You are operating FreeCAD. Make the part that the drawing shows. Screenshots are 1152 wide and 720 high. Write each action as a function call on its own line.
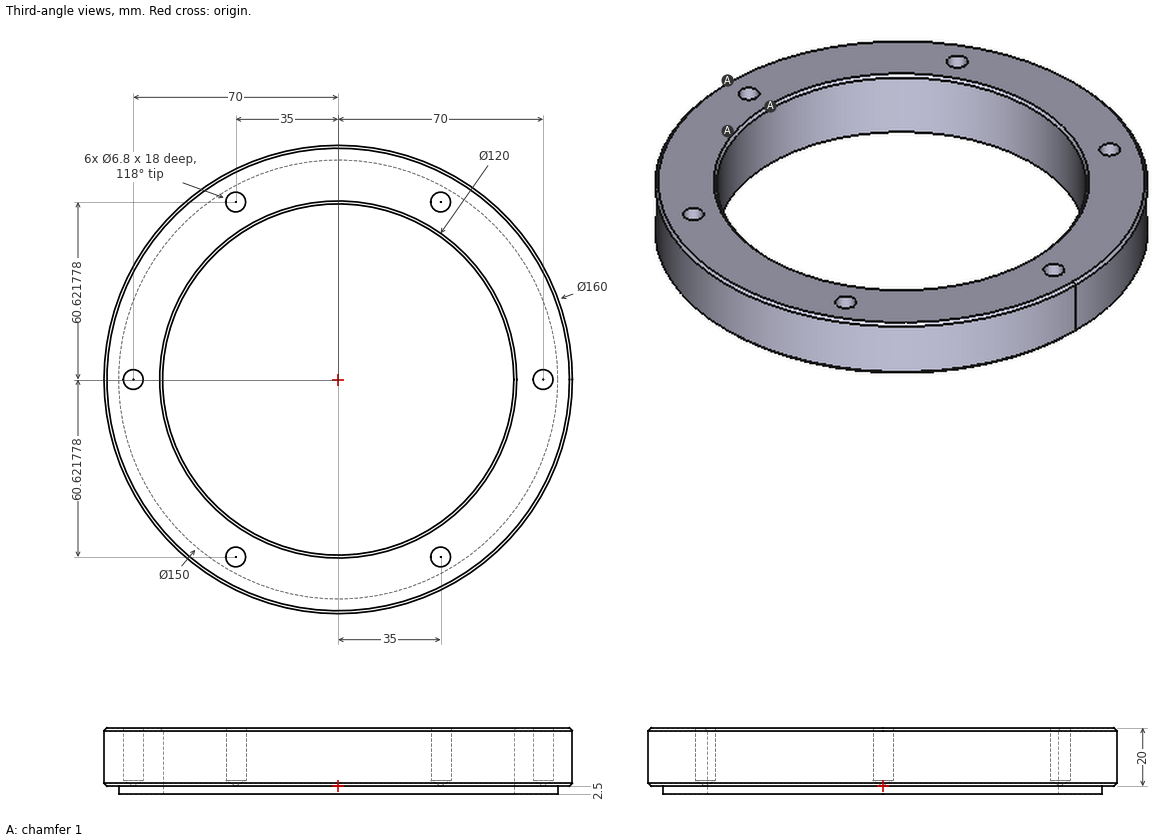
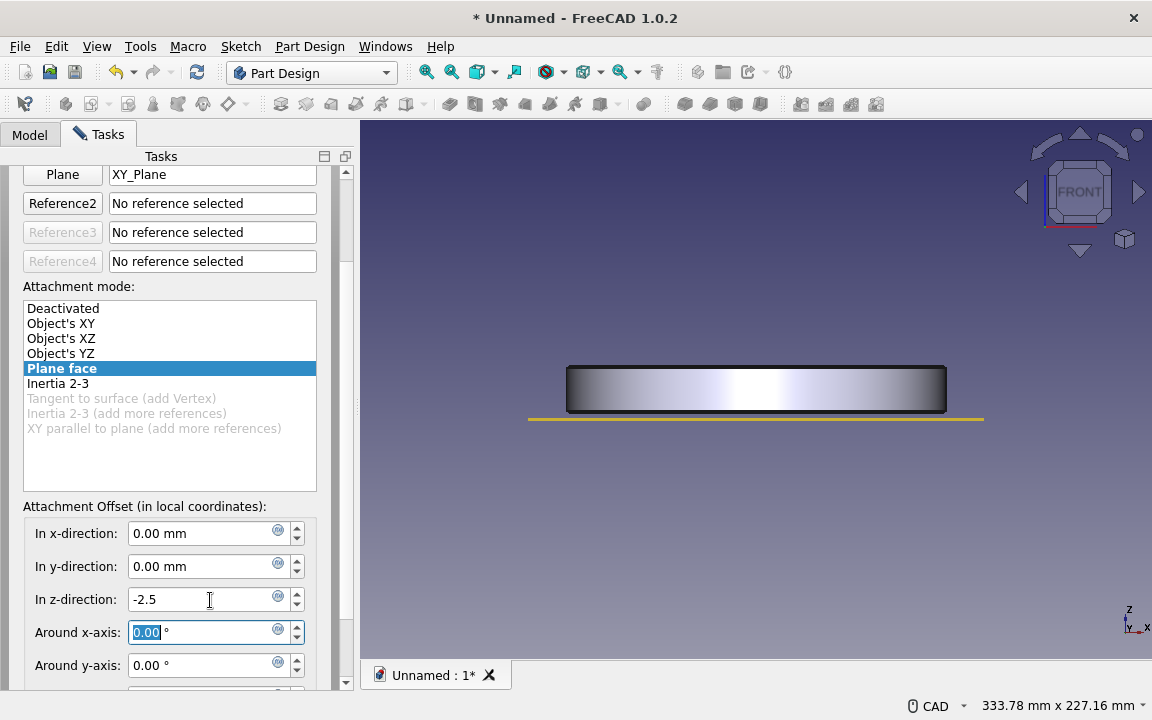
scroll(346, 428, up, 3)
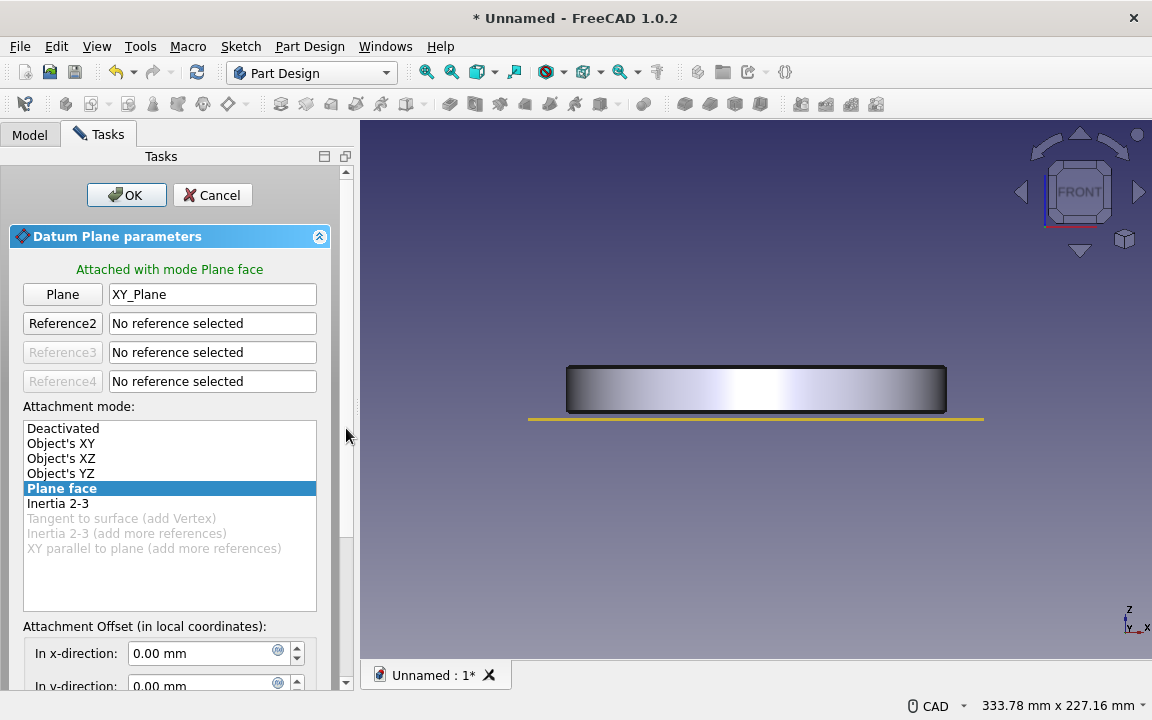
click(127, 195)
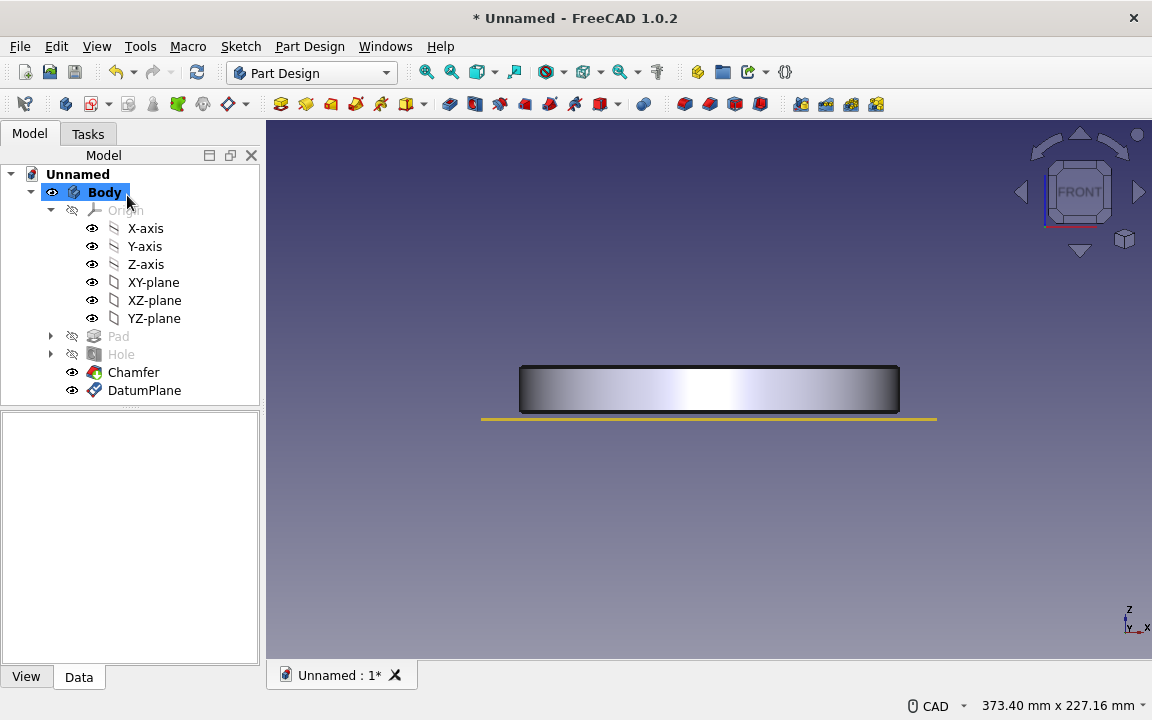
click(117, 390)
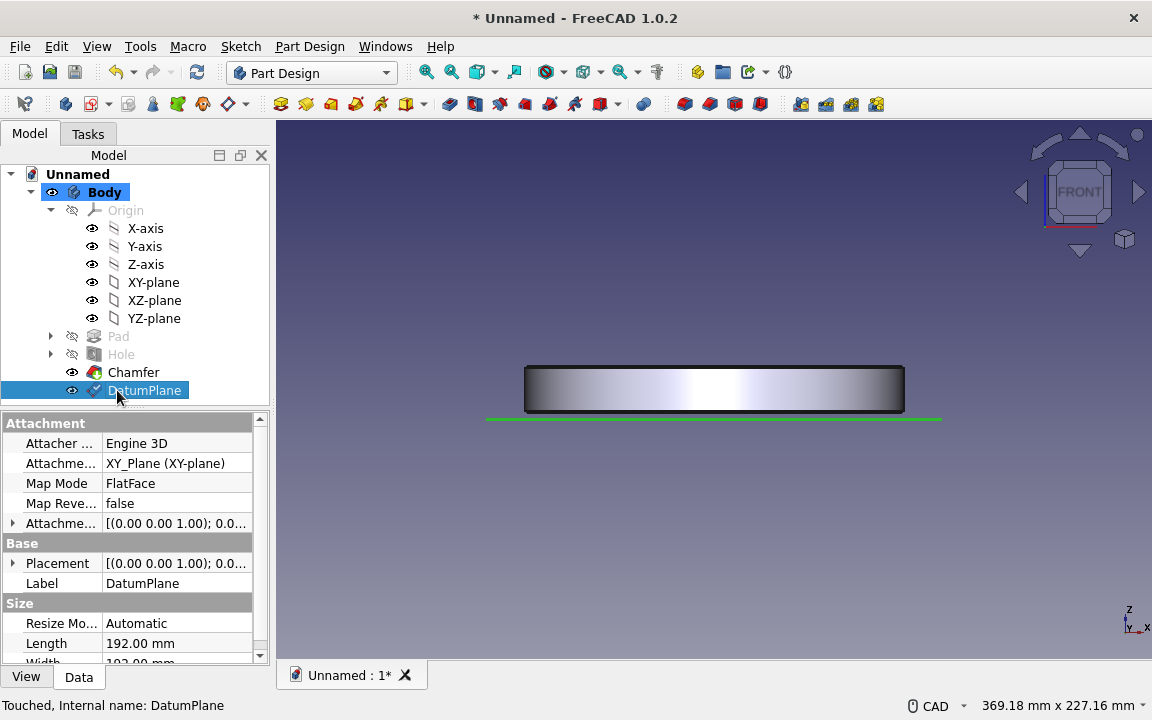
click(90, 104)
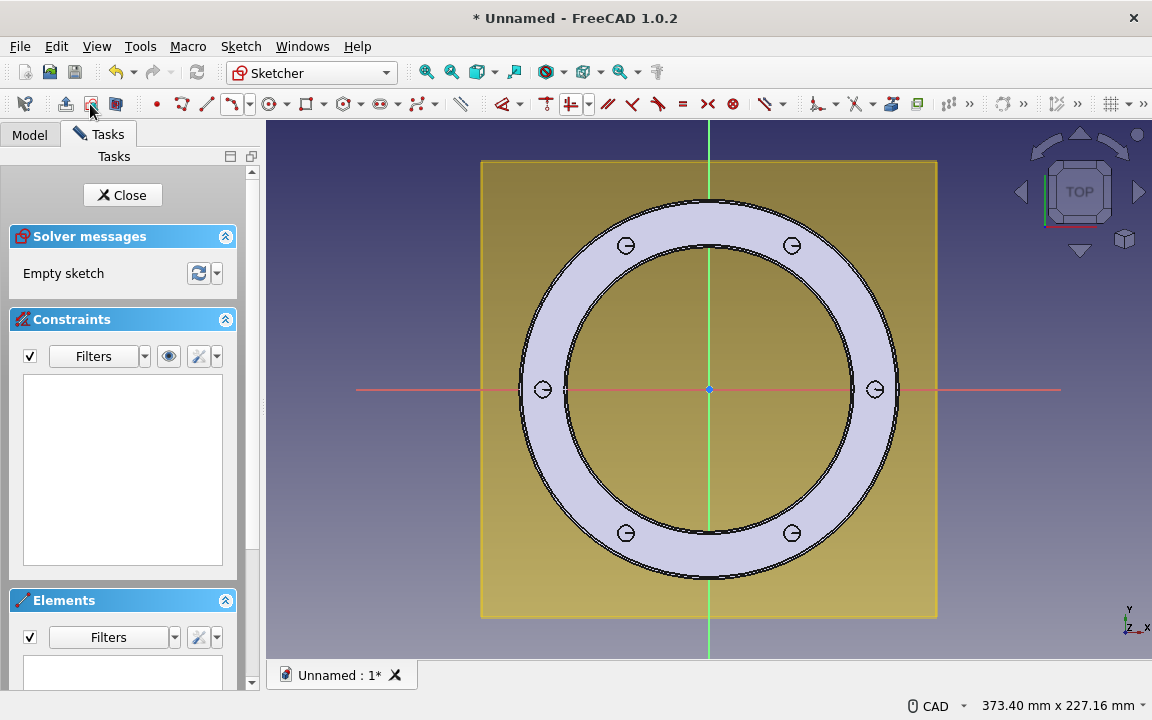
click(116, 104)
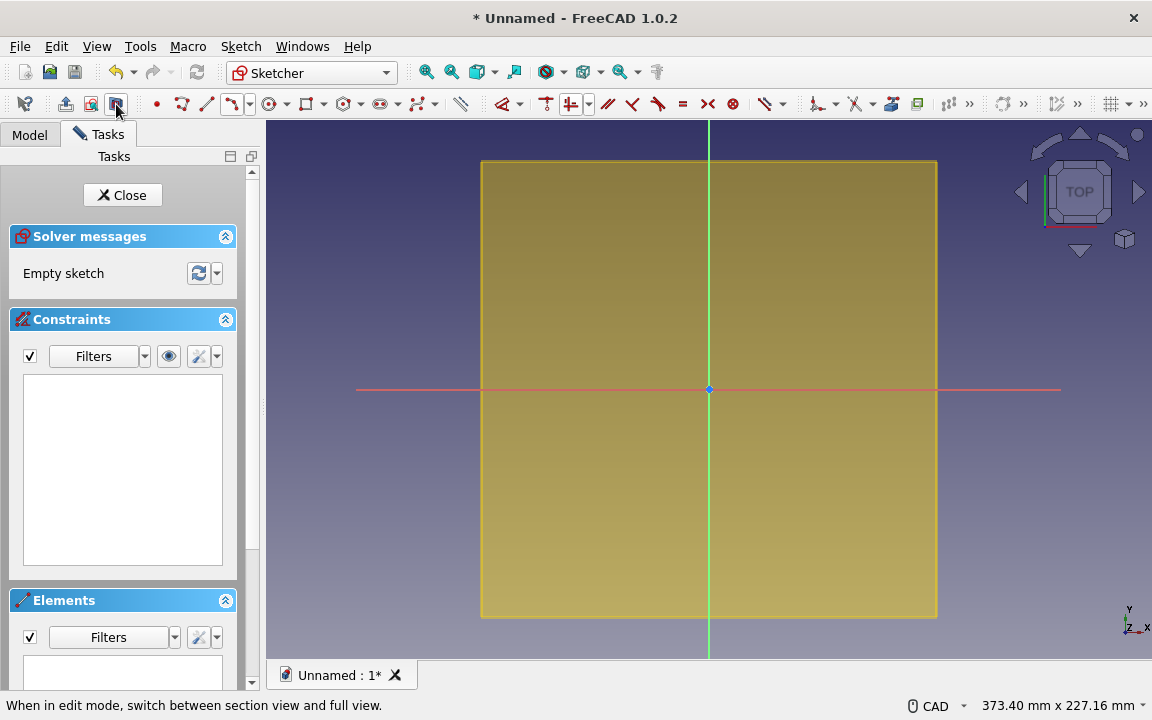
key(g)
key(c)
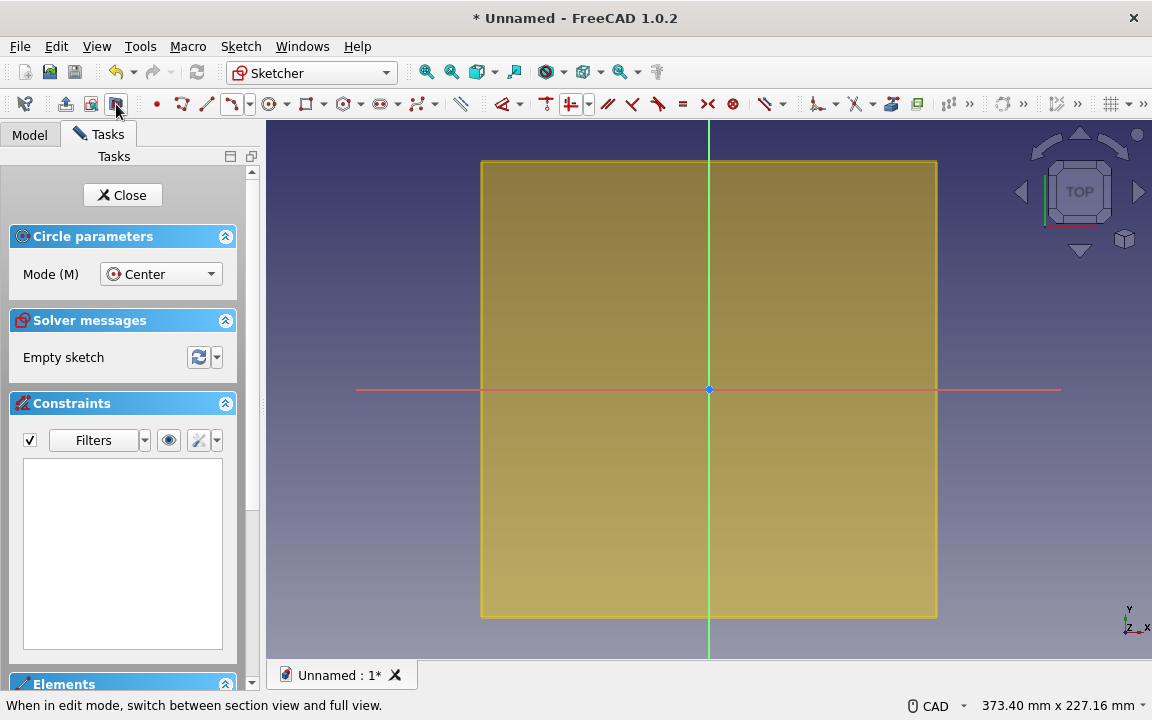
click(709, 390)
click(835, 264)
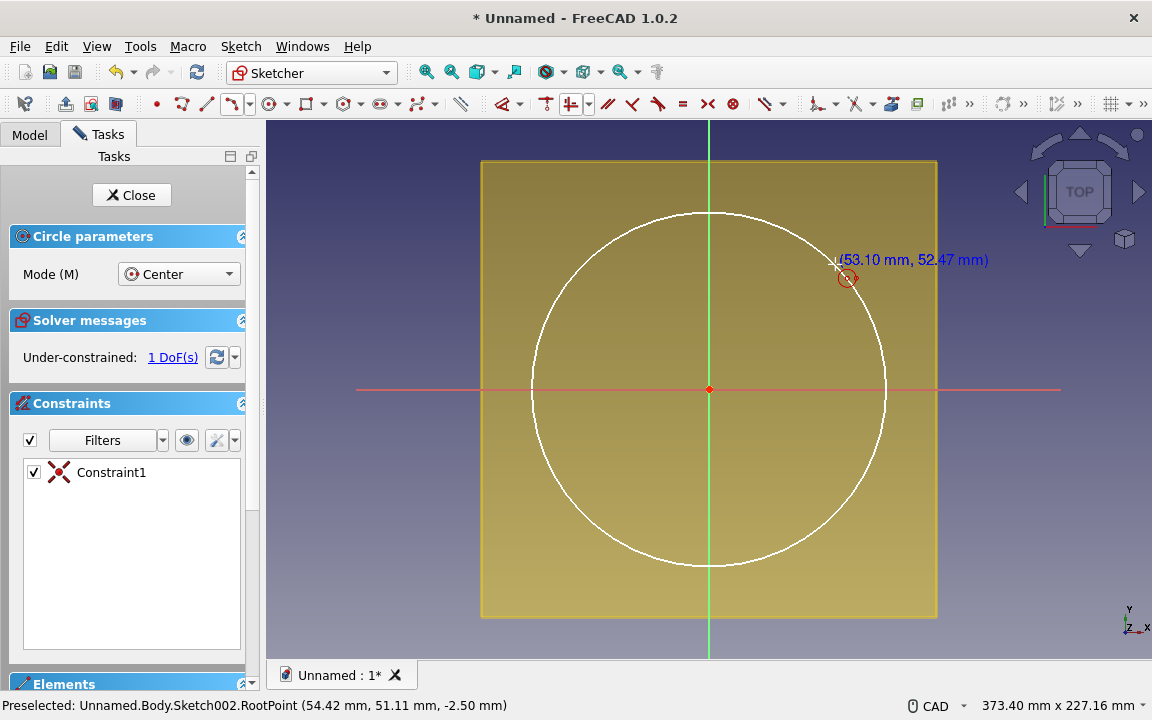
click(709, 390)
click(810, 289)
key(Escape)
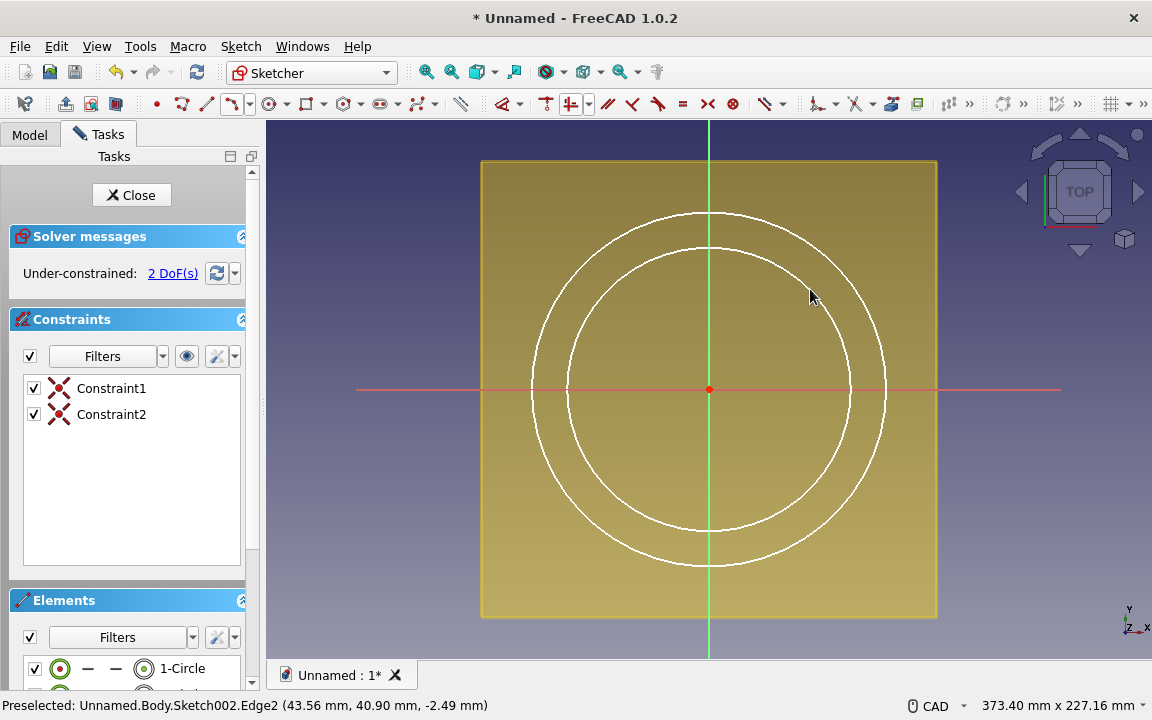
click(502, 104)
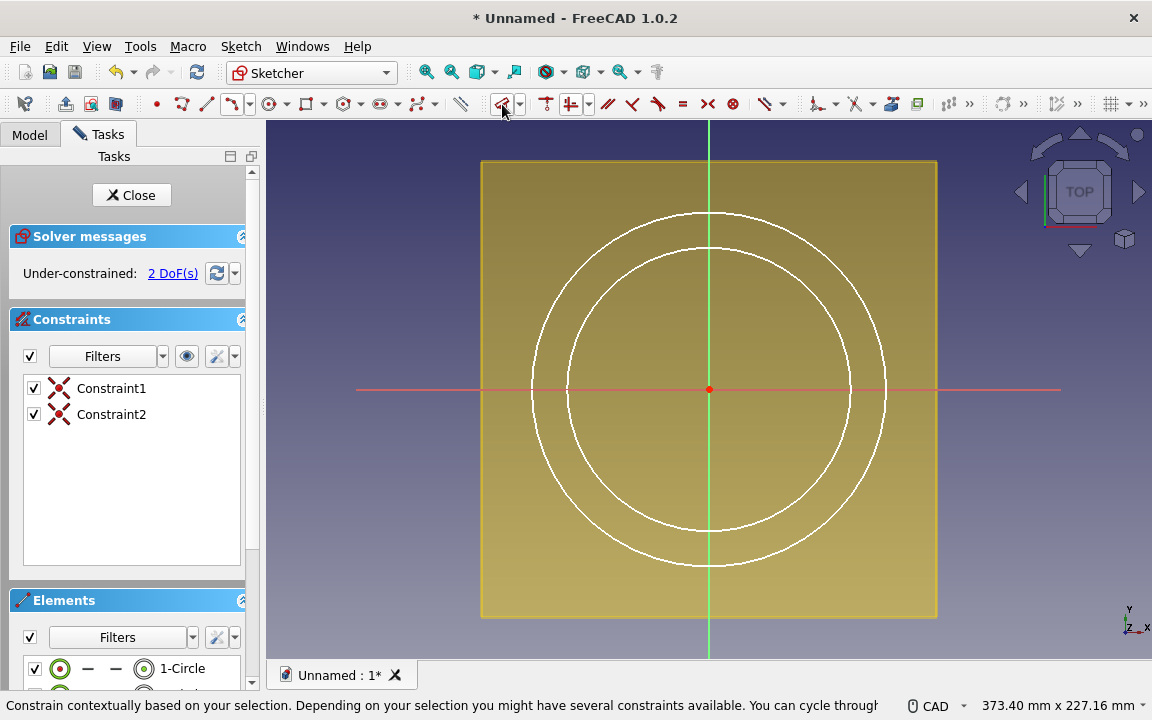
click(834, 264)
click(857, 241)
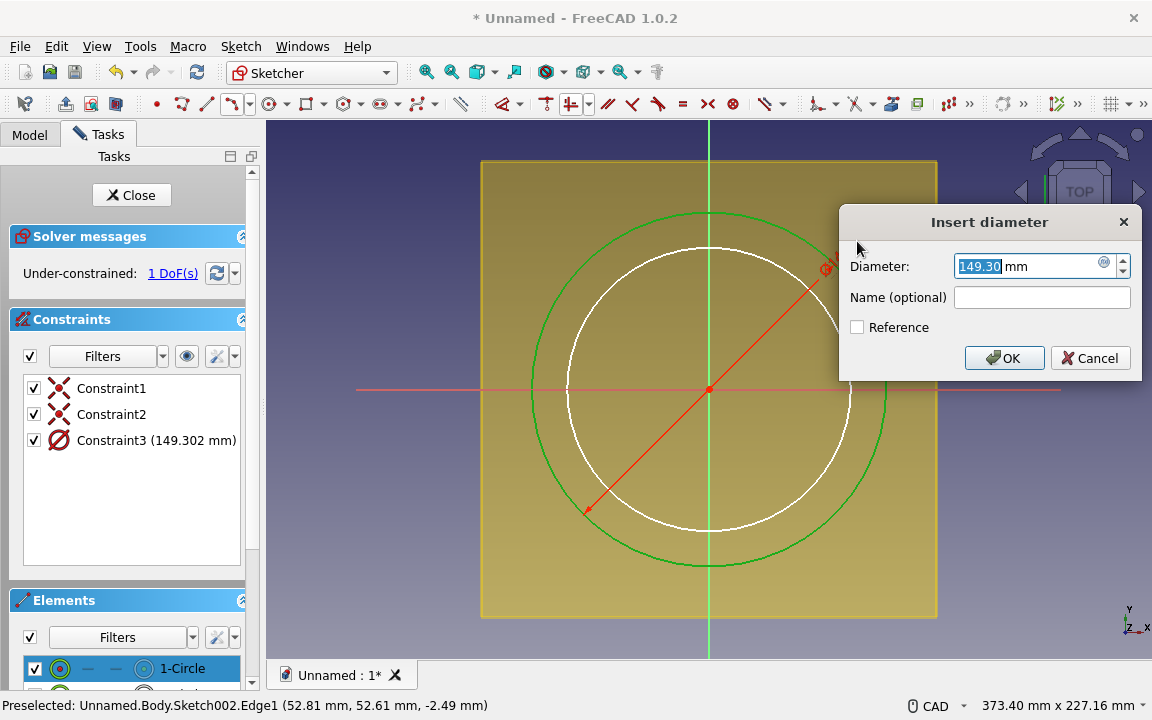
text(150)
key(Return)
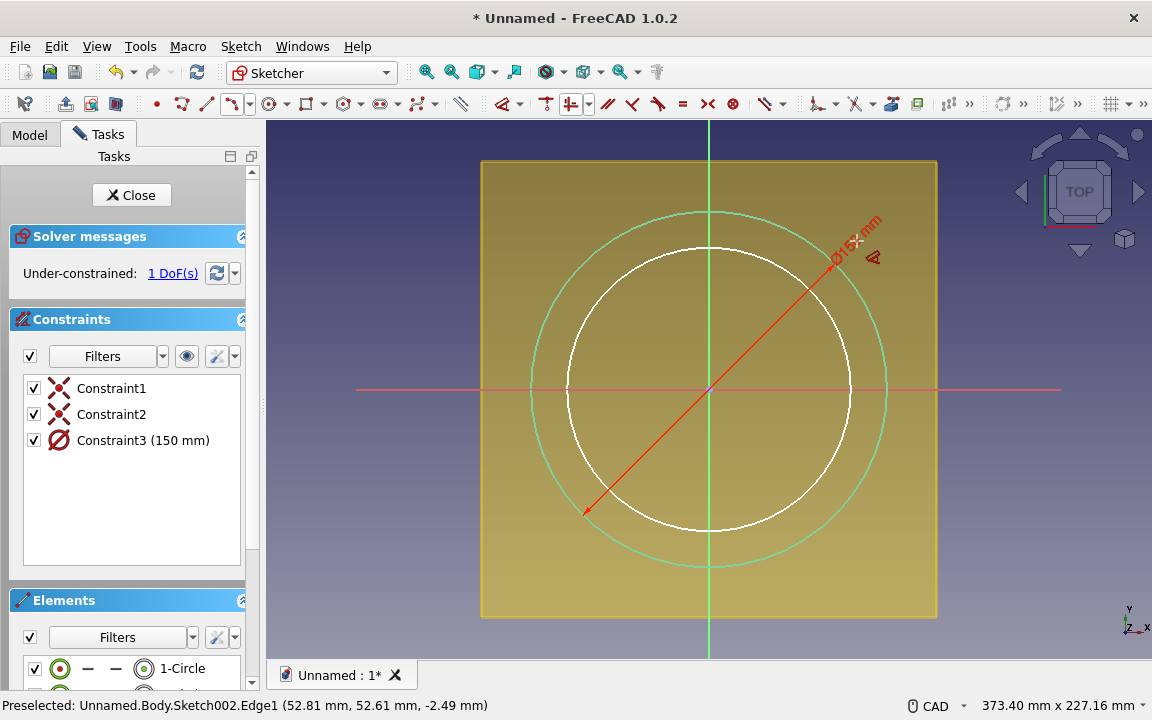
click(809, 289)
click(898, 334)